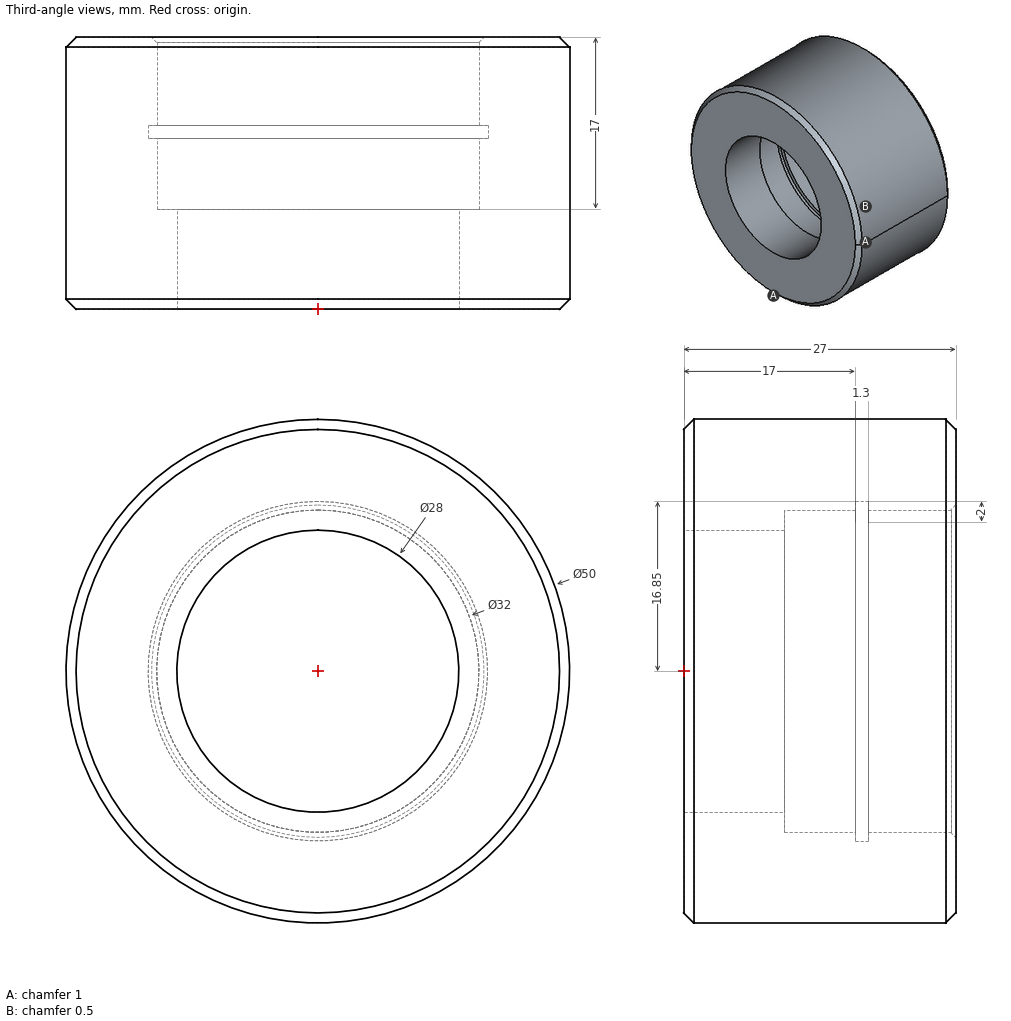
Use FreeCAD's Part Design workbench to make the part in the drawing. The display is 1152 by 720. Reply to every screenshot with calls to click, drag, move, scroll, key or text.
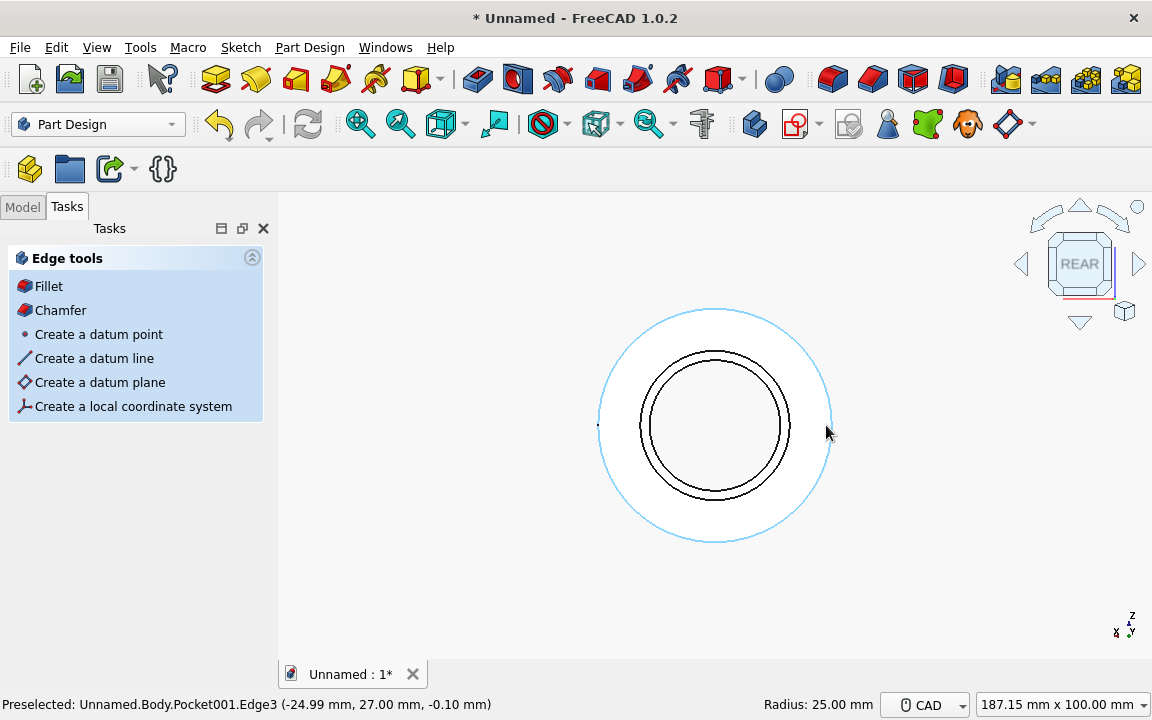
key(0)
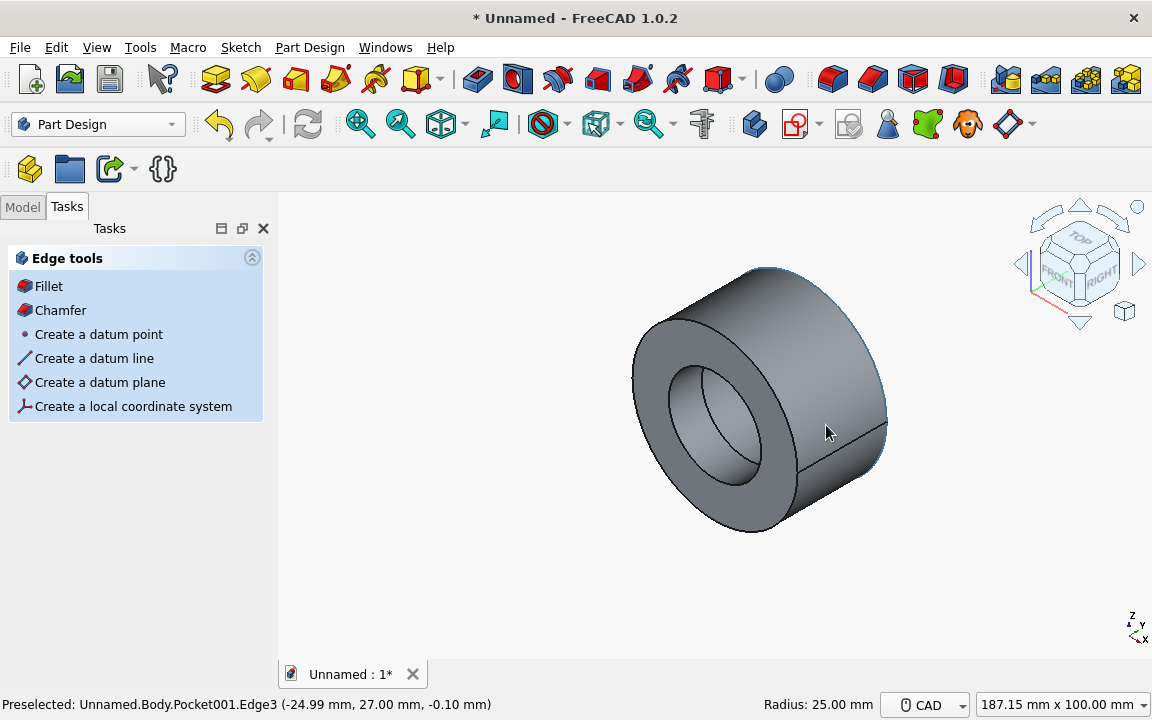
click(689, 319, ctrl)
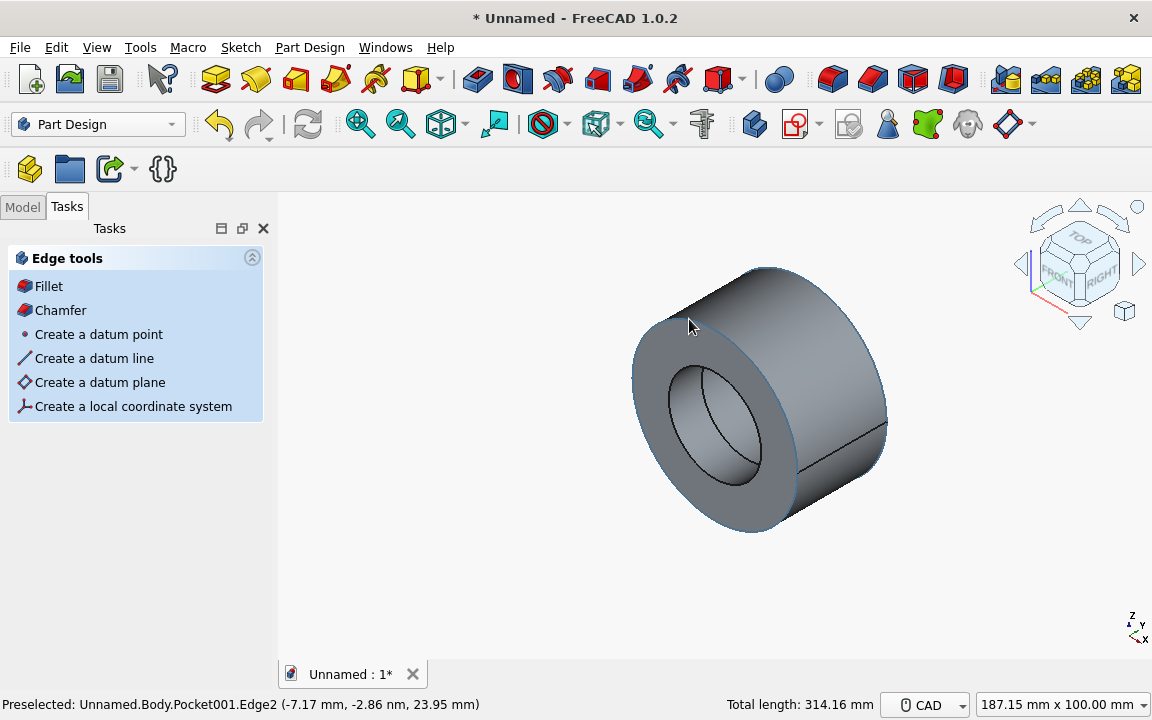
click(874, 80)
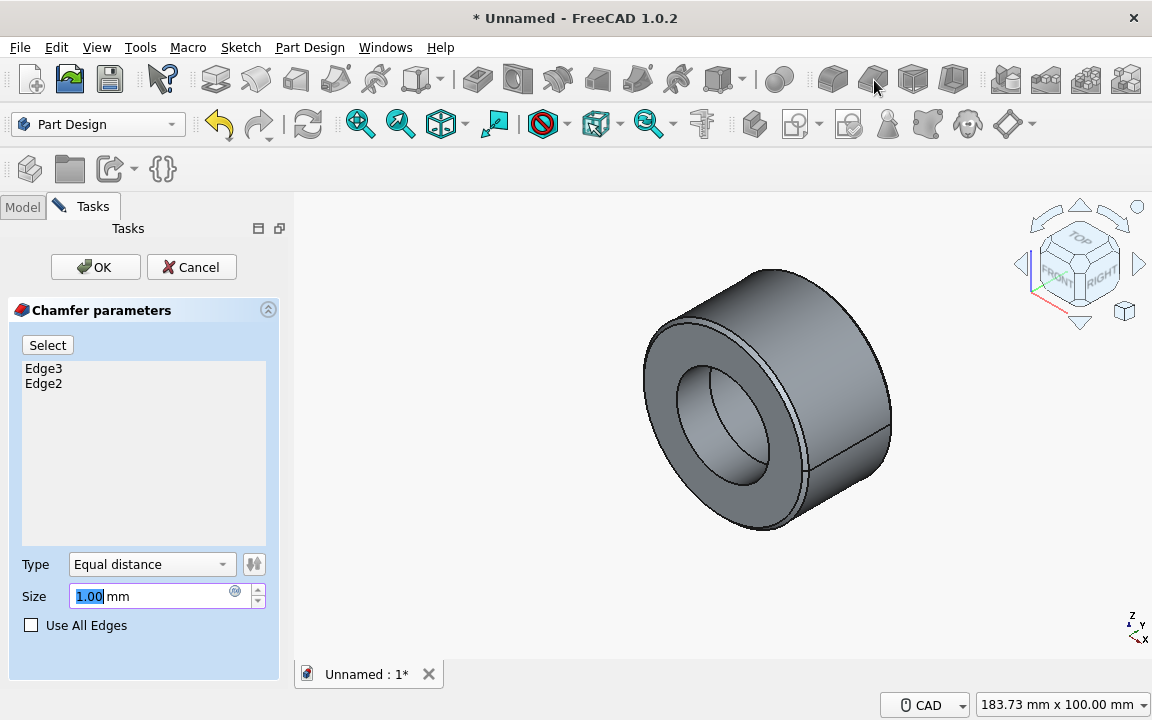
text(1)
key(Tab)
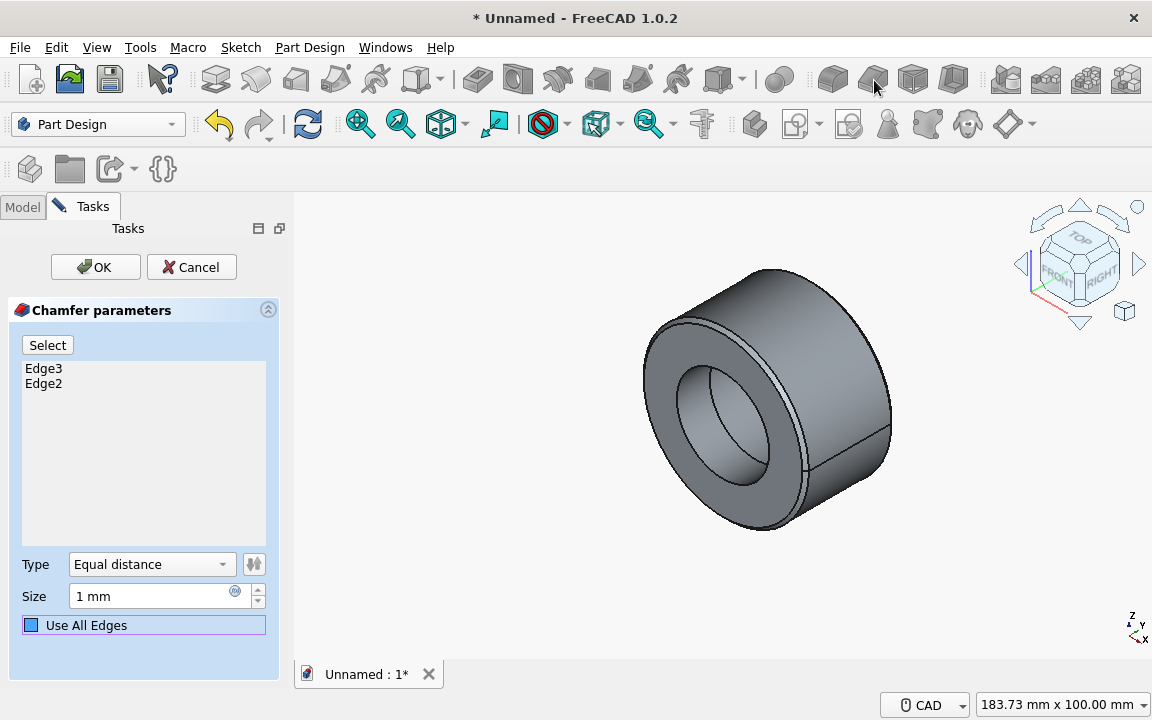
click(96, 267)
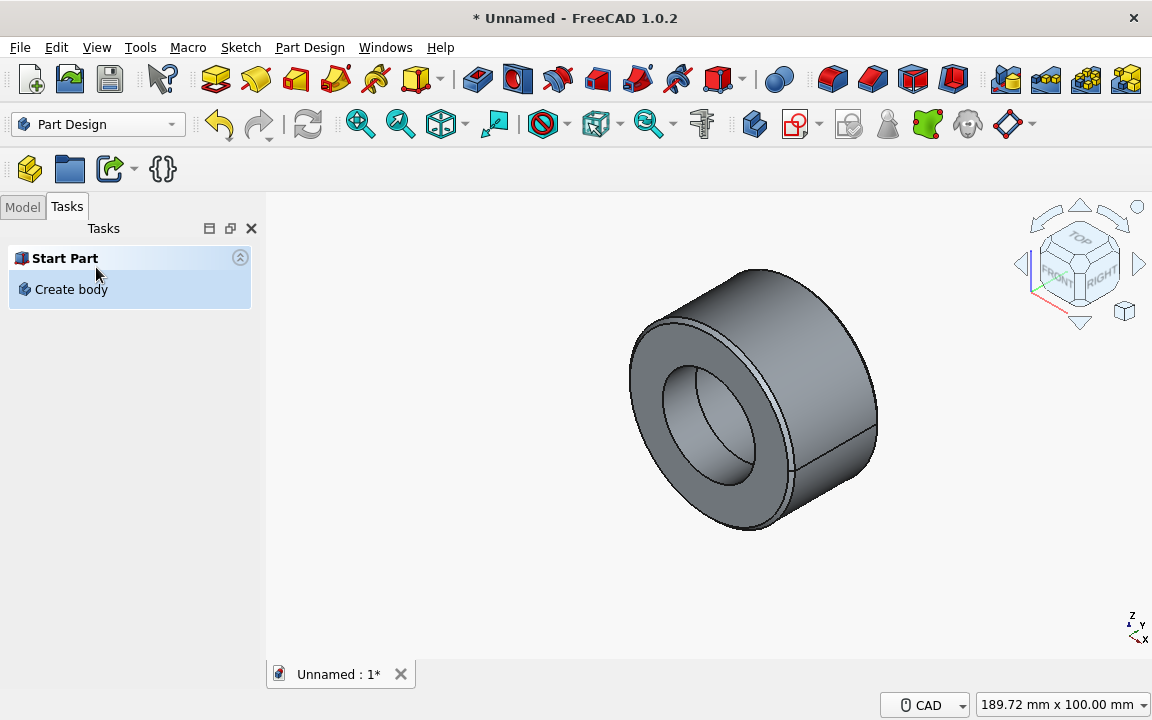
key(2)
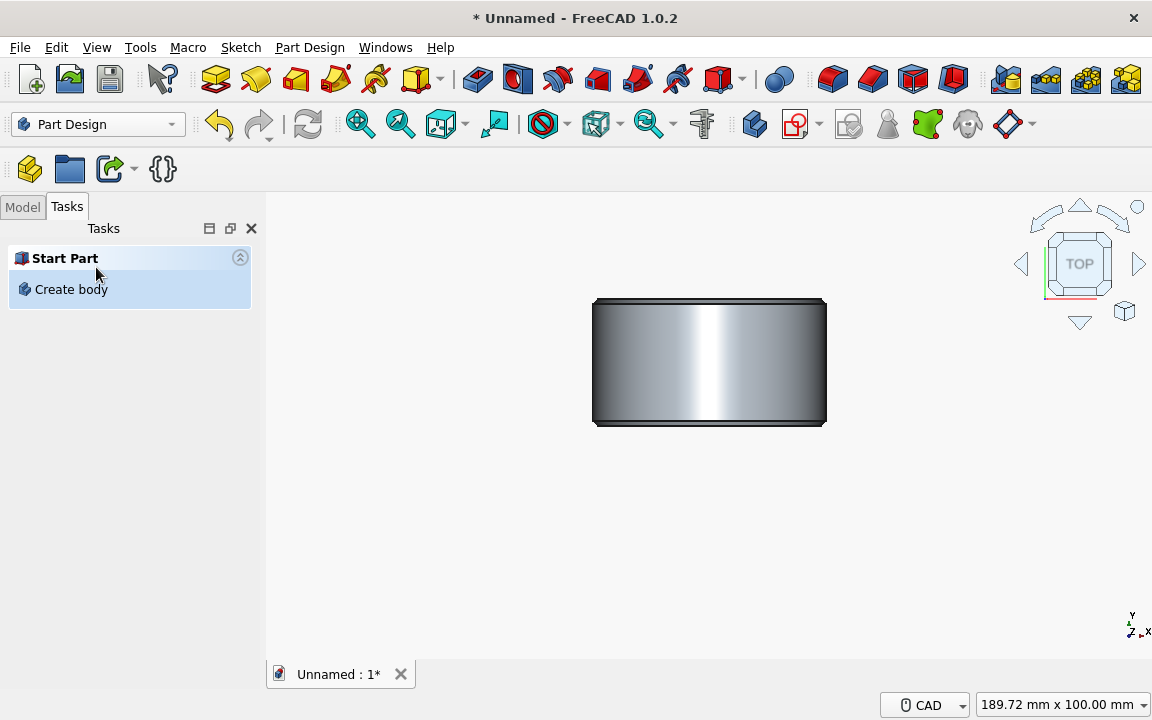
key(v)
key(f)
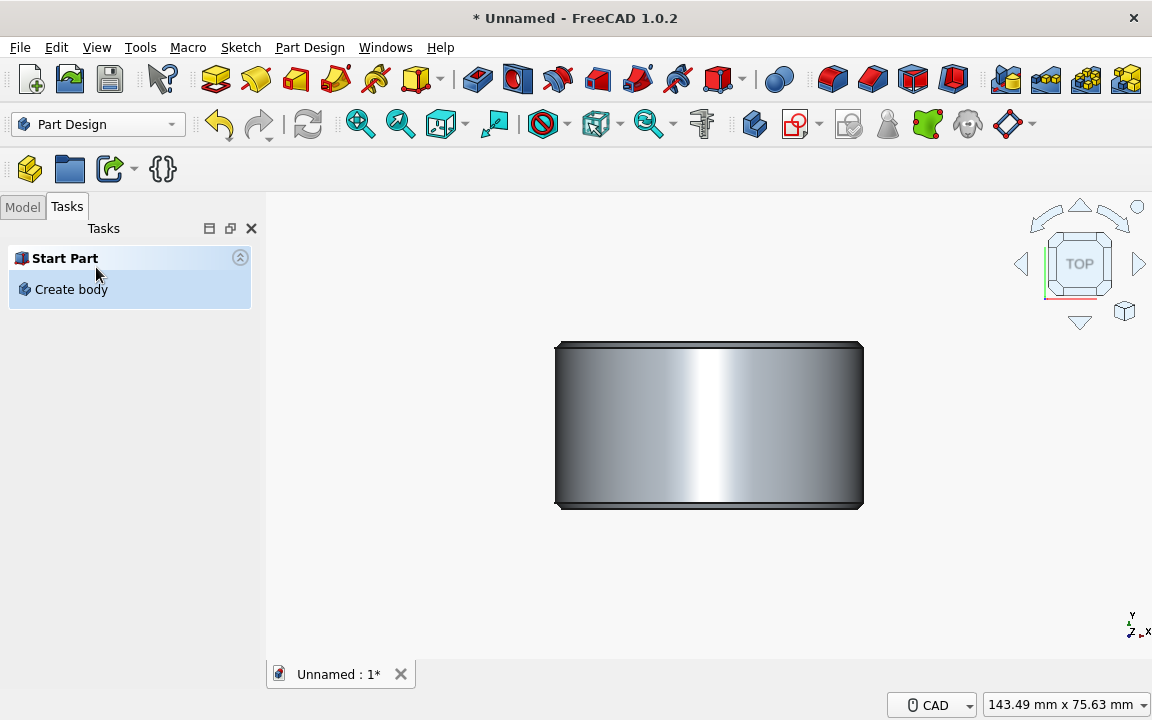
key(0)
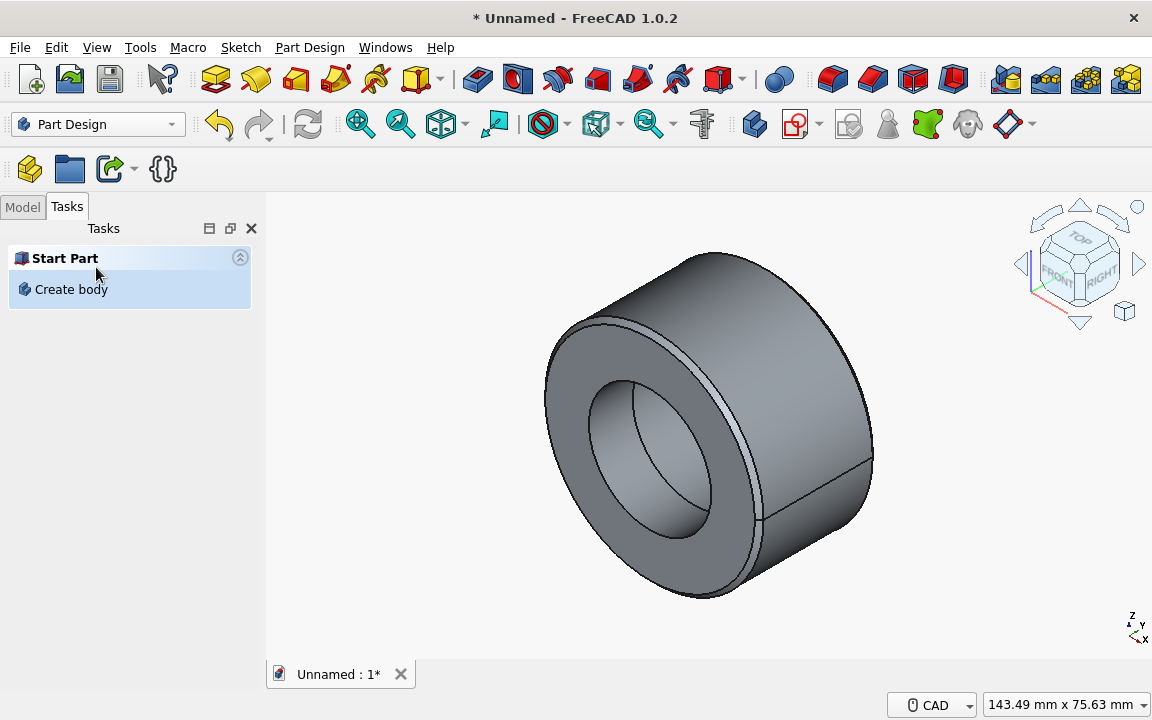
key(1)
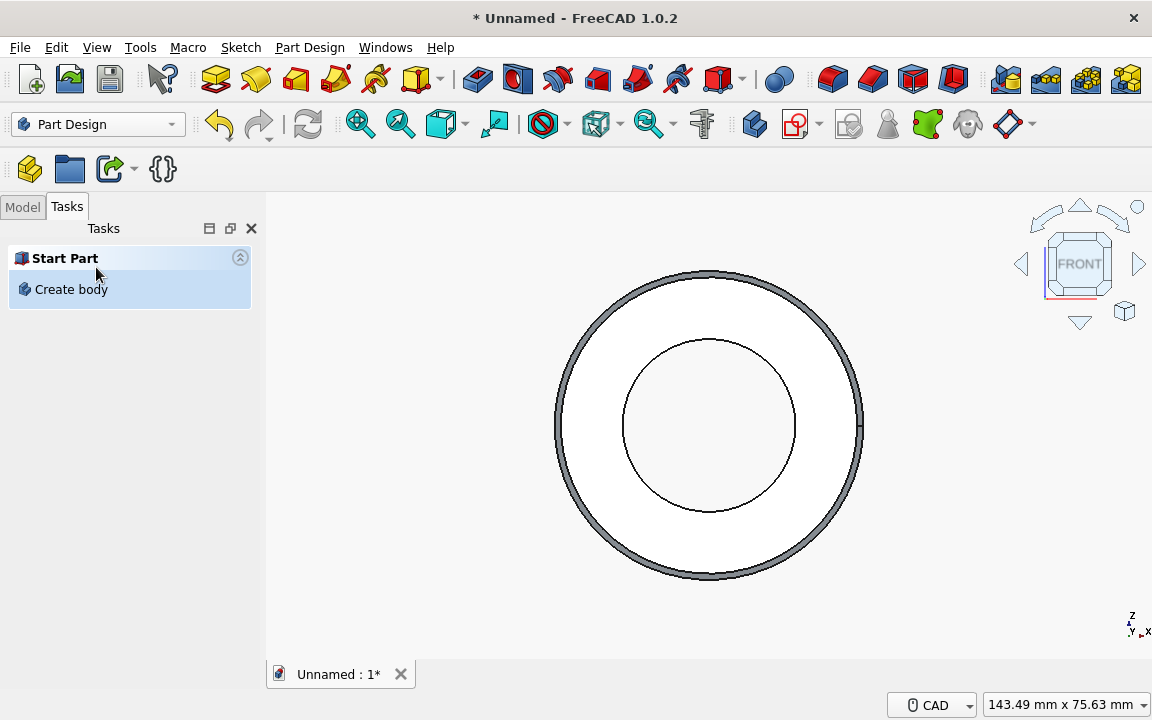
key(3)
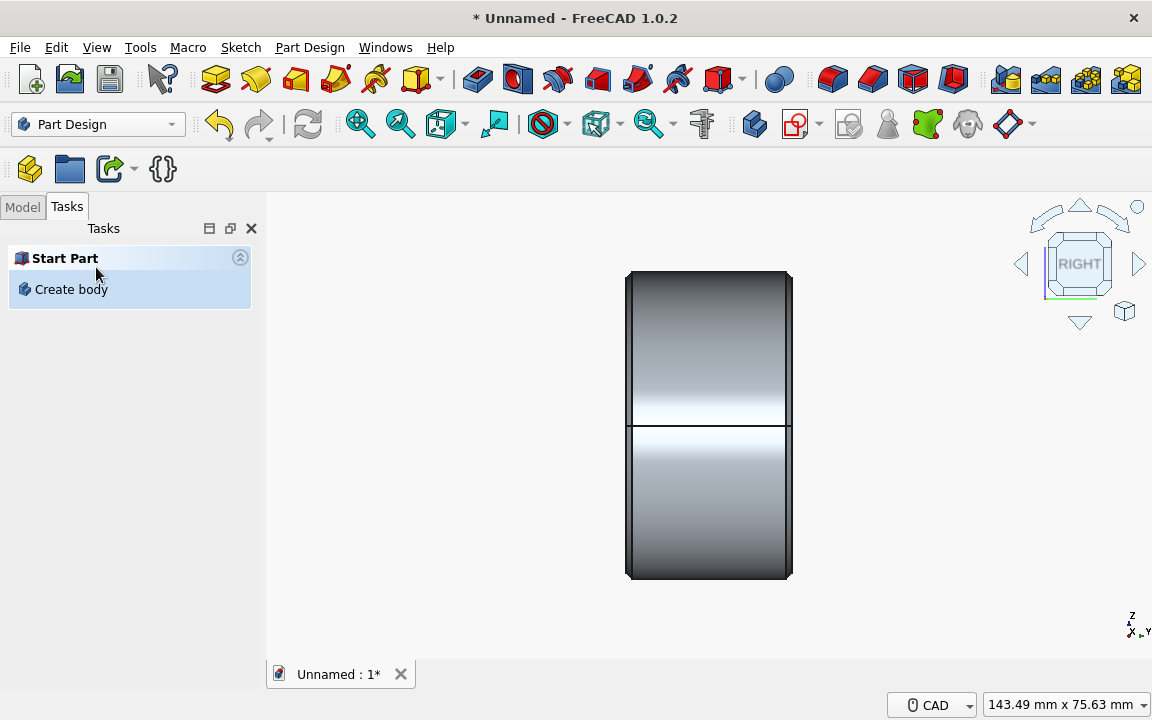
key(5)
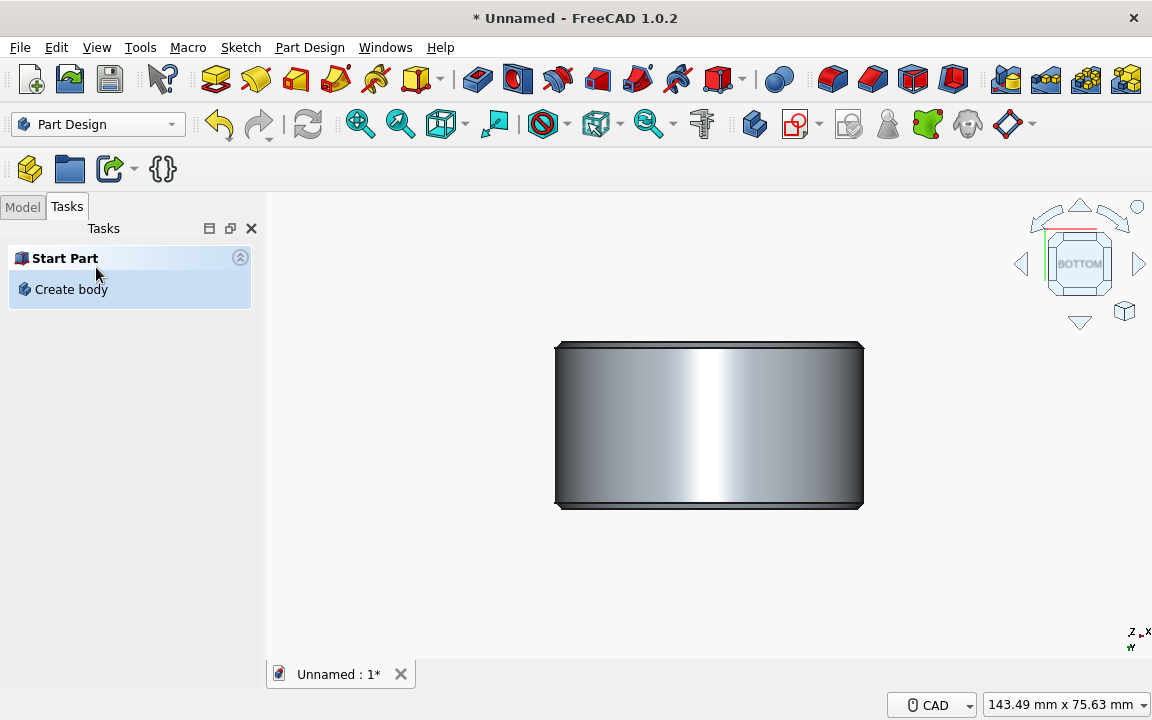
click(362, 124)